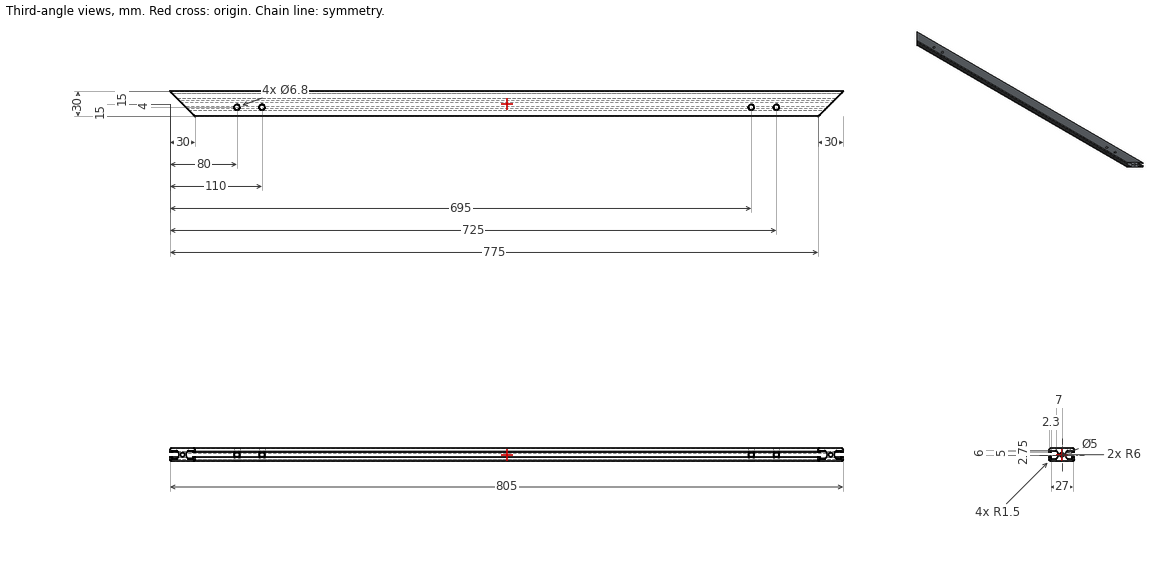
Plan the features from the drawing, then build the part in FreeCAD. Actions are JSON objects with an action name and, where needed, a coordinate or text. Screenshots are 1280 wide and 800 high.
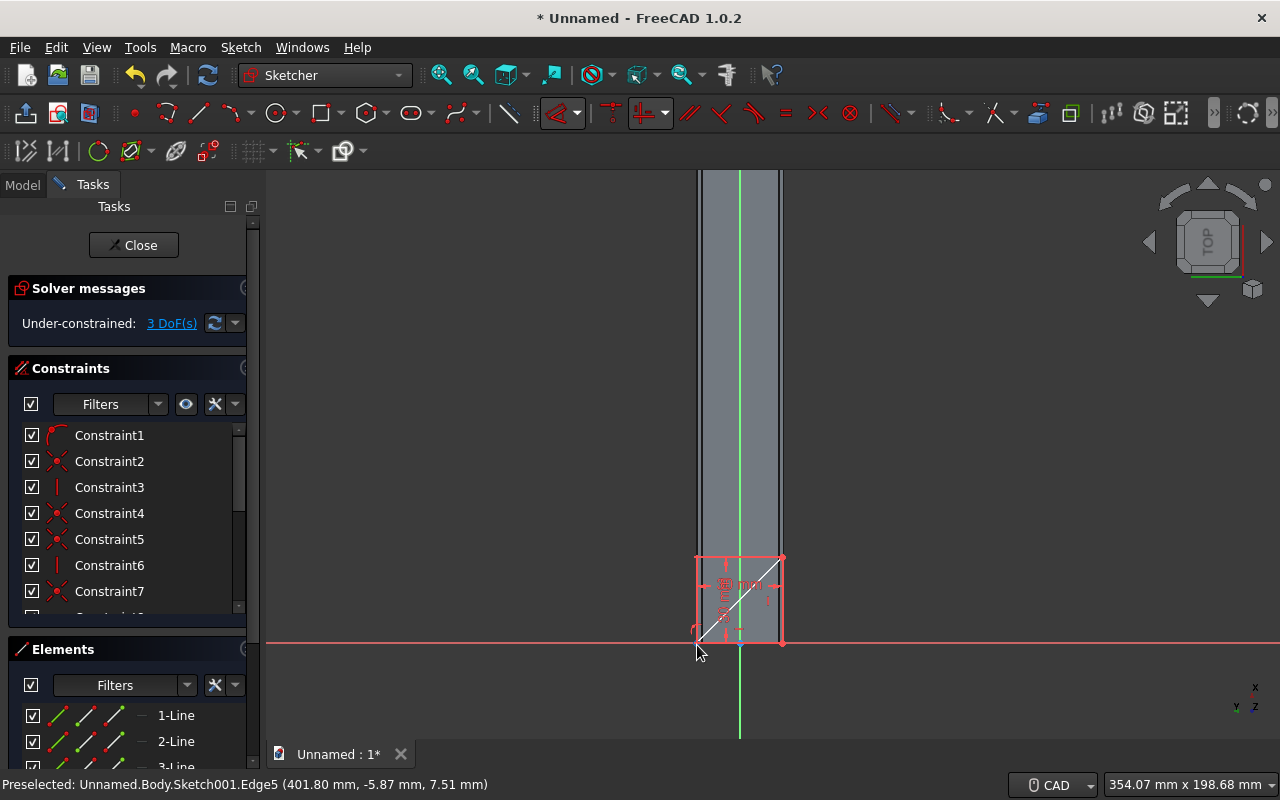
{"action": "left_click", "coordinate": [697, 643]}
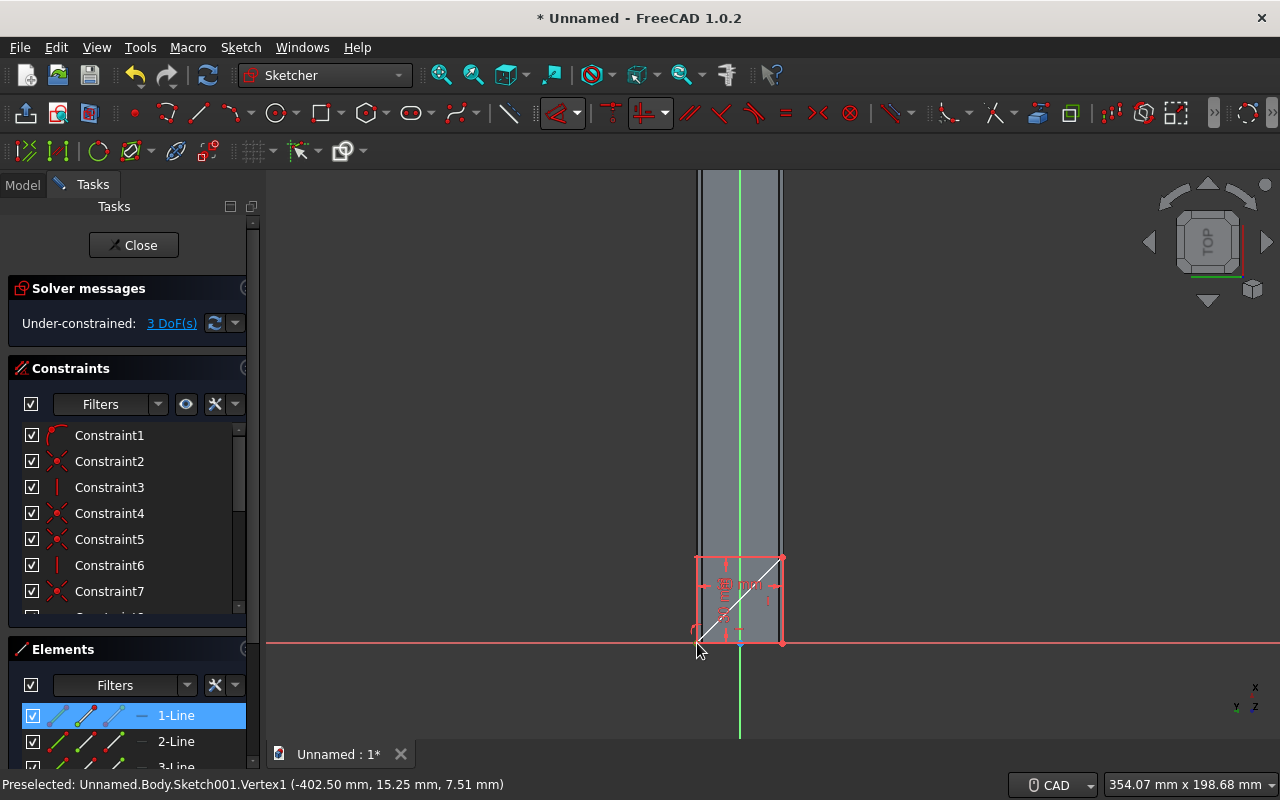
{"action": "key", "text": "l"}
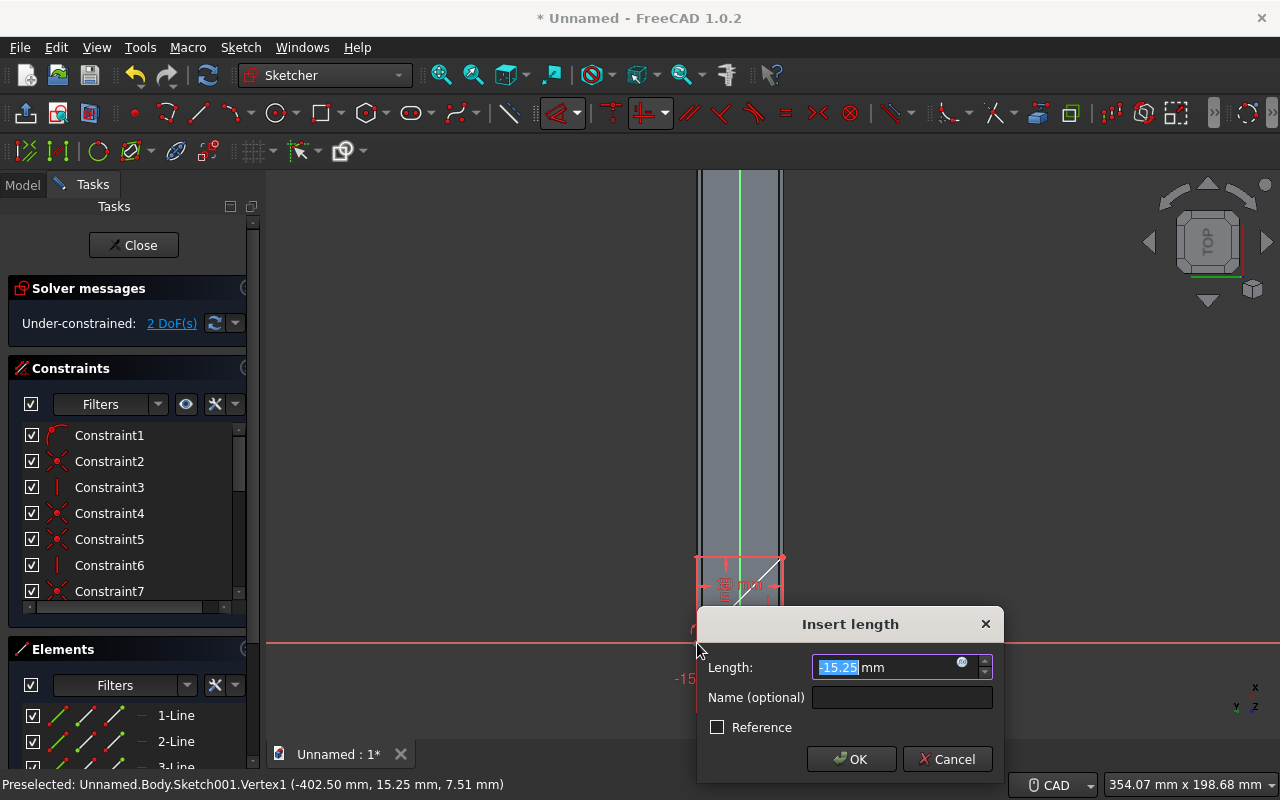
{"action": "type", "text": "-15"}
{"action": "key", "text": "Return"}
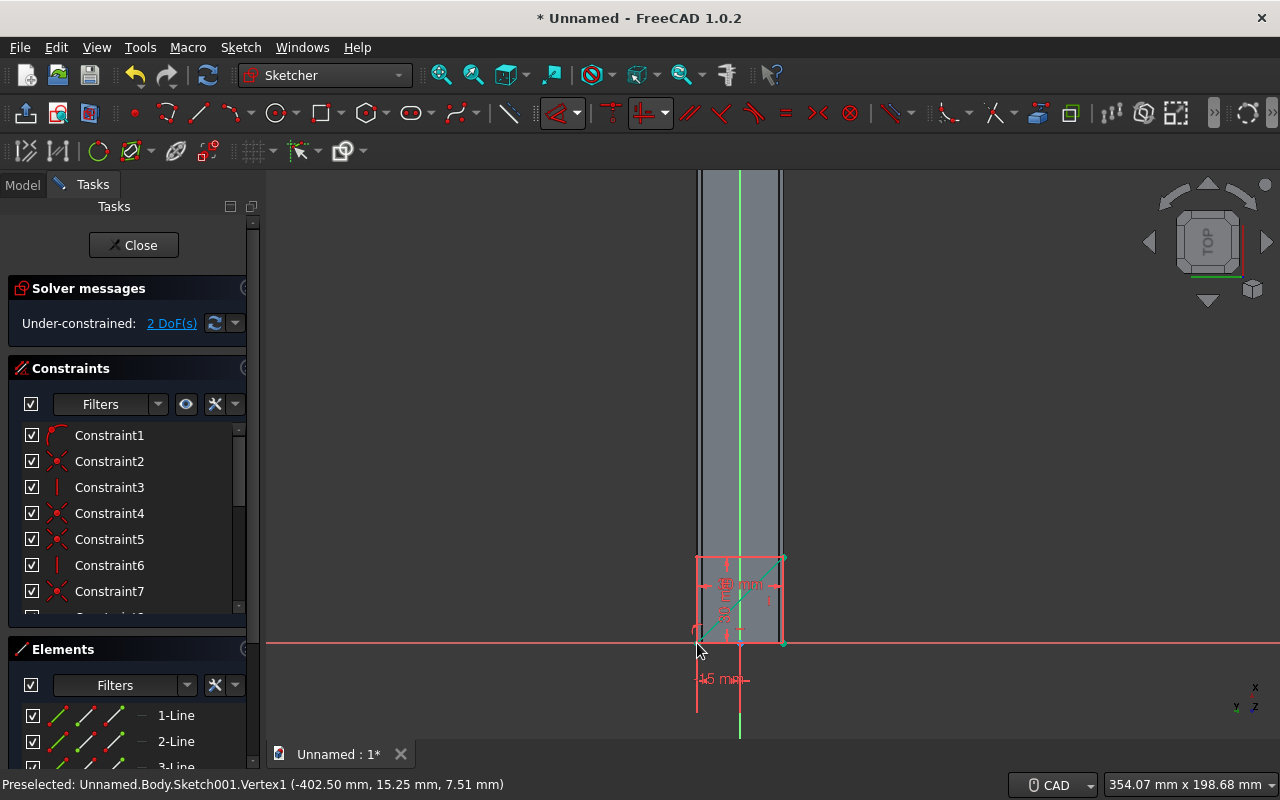
{"action": "scroll", "coordinate": [697, 645], "scroll_direction": "down", "scroll_amount": 9}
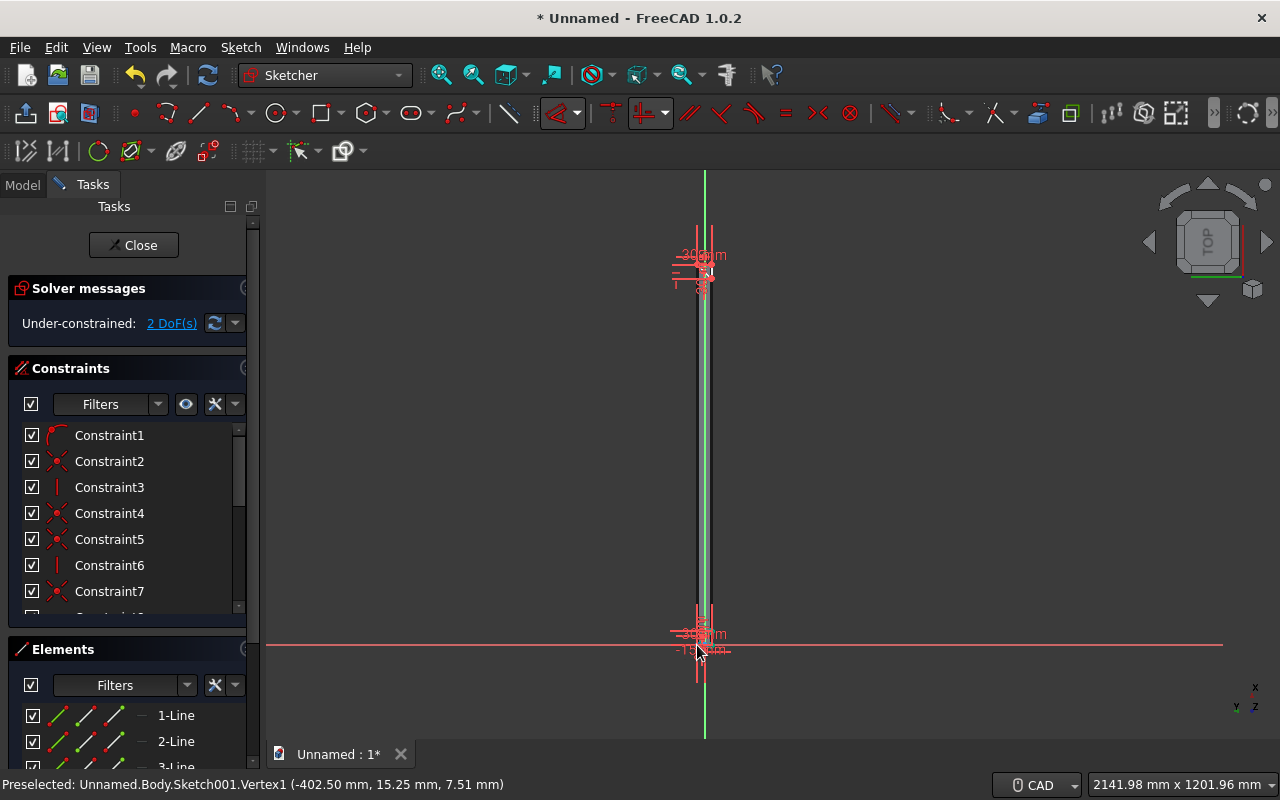
{"action": "scroll", "coordinate": [712, 279], "scroll_direction": "up", "scroll_amount": 9}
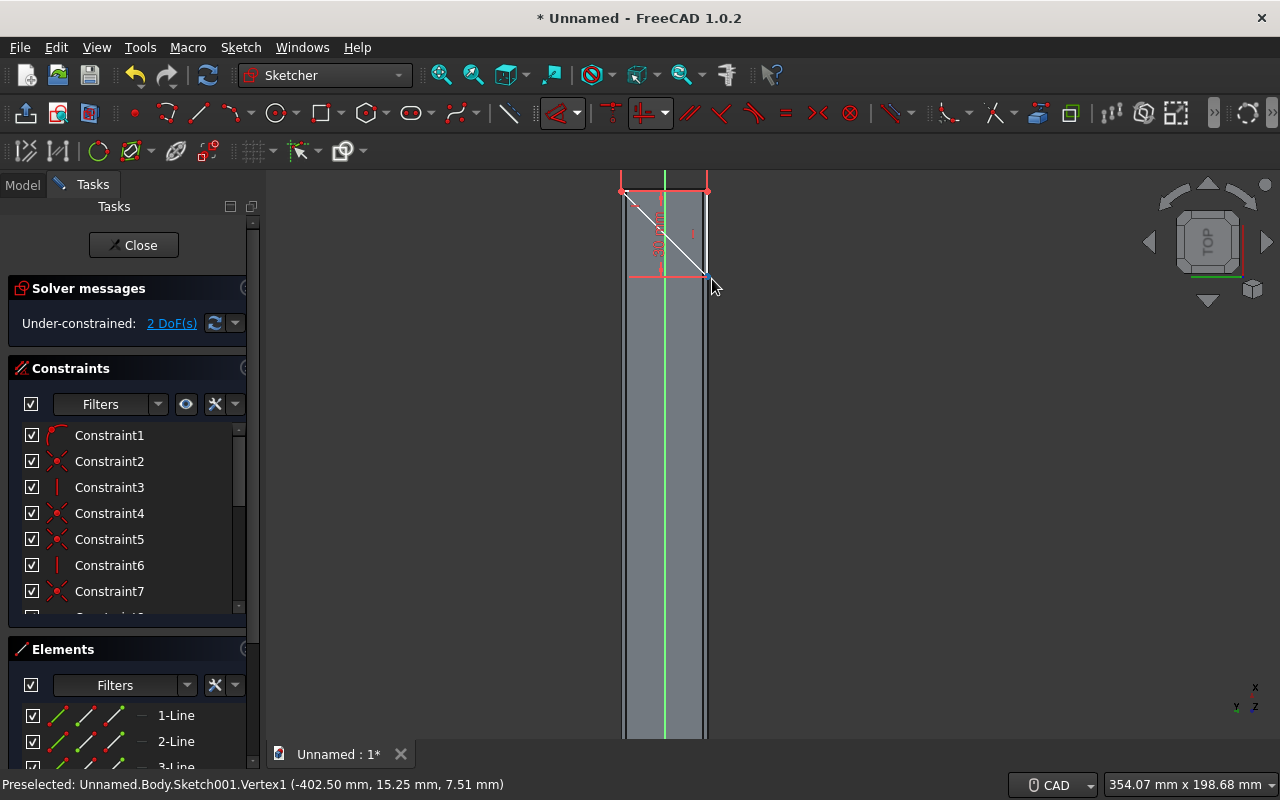
{"action": "left_click", "coordinate": [707, 277]}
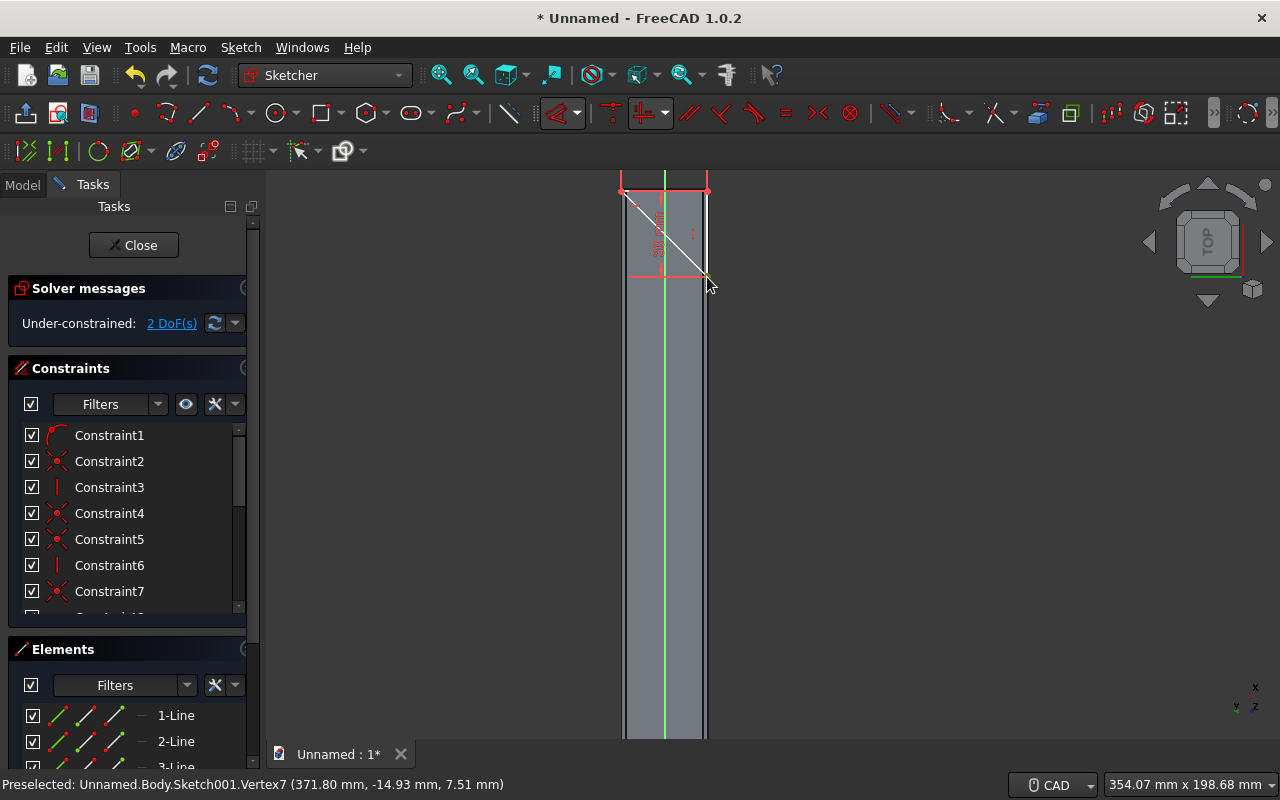
{"action": "key", "text": "l"}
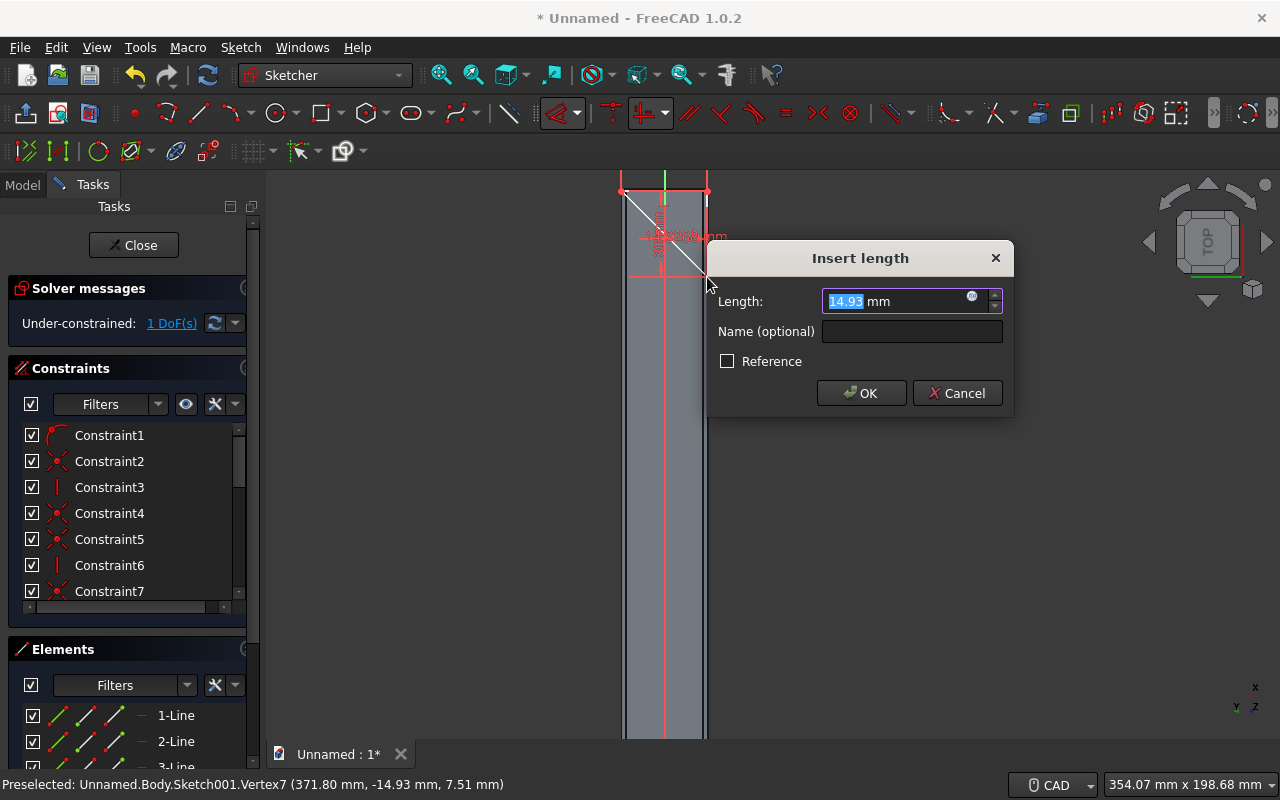
{"action": "type", "text": "15"}
{"action": "key", "text": "Return"}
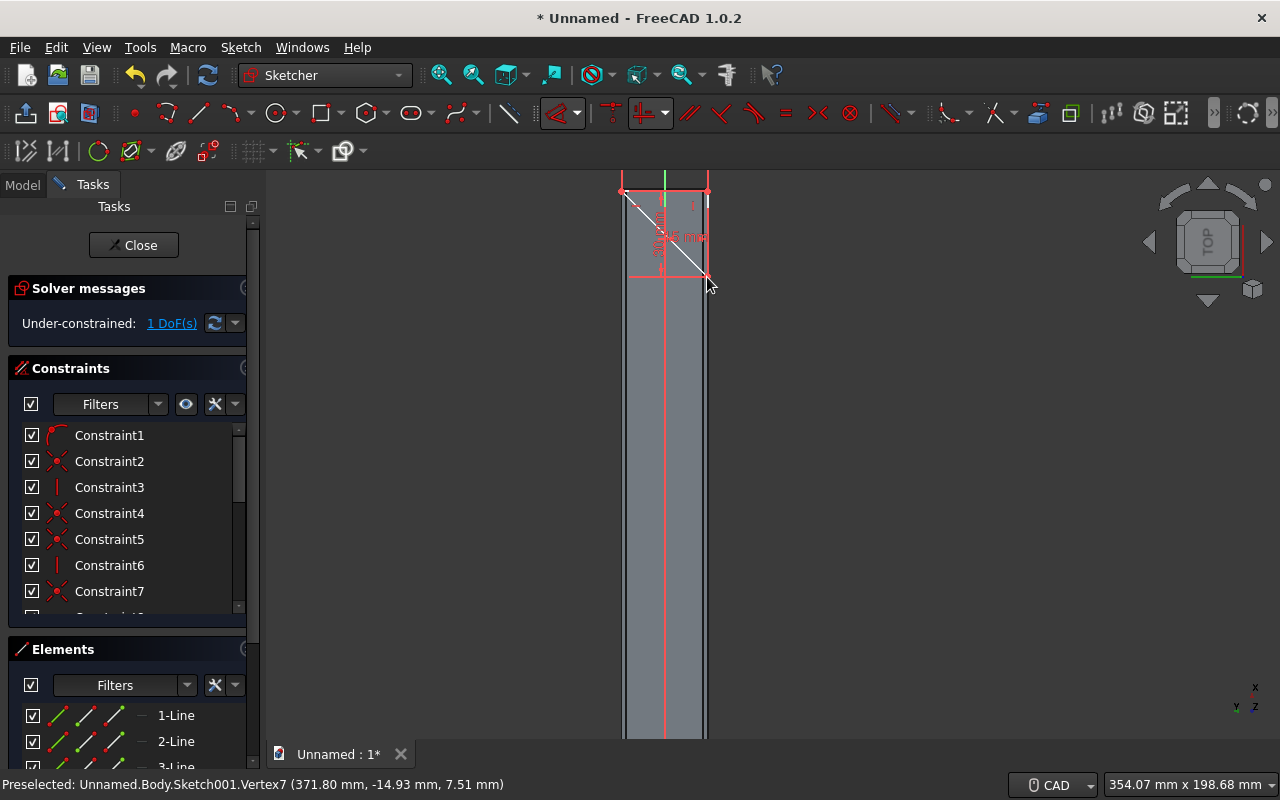
{"action": "scroll", "coordinate": [712, 279], "scroll_direction": "down", "scroll_amount": 9}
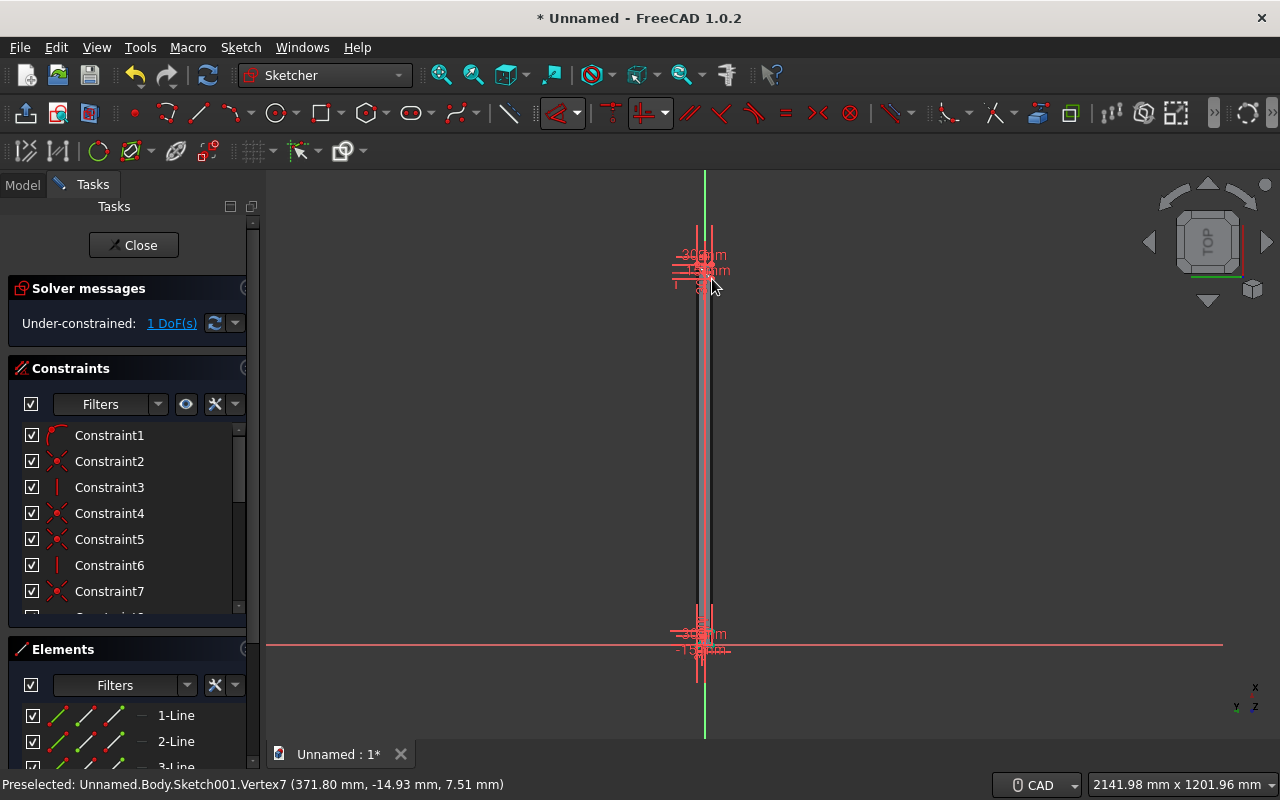
{"action": "left_click", "coordinate": [712, 279]}